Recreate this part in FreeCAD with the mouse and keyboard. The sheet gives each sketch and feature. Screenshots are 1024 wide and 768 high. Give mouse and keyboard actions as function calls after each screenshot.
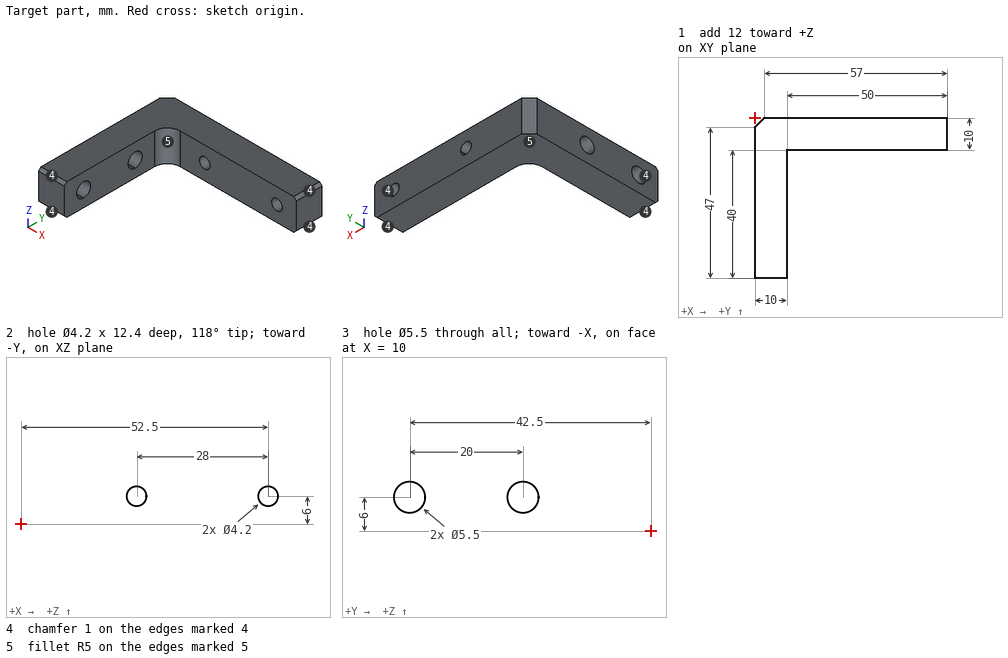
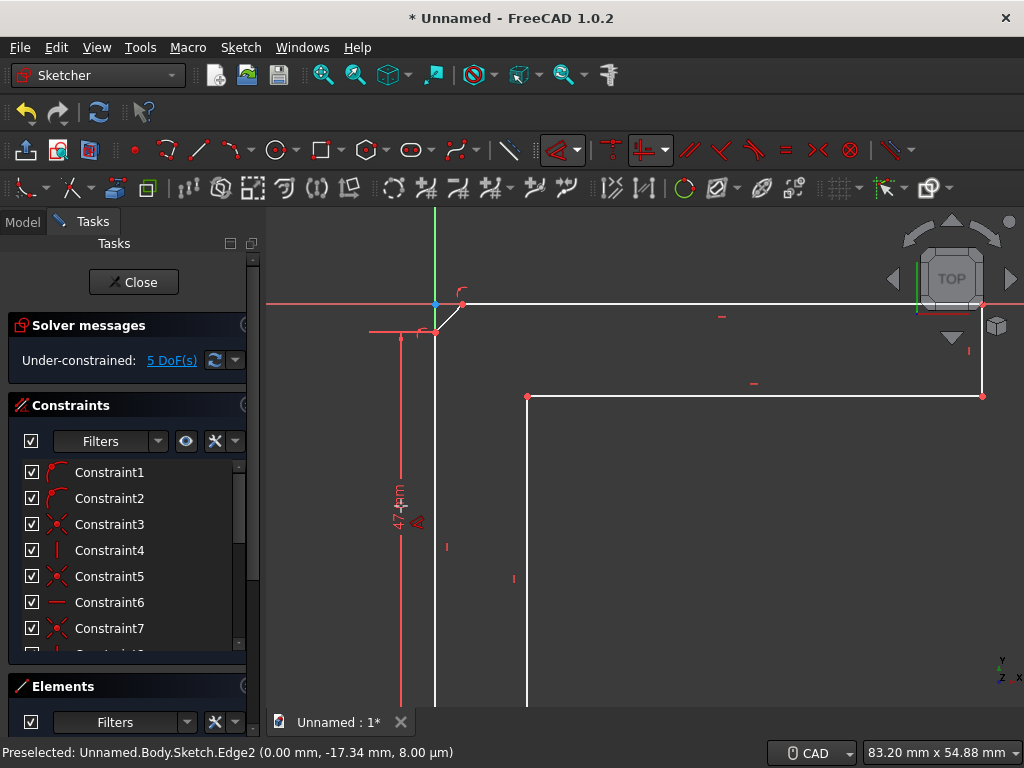
scroll(308, 305, down, 2)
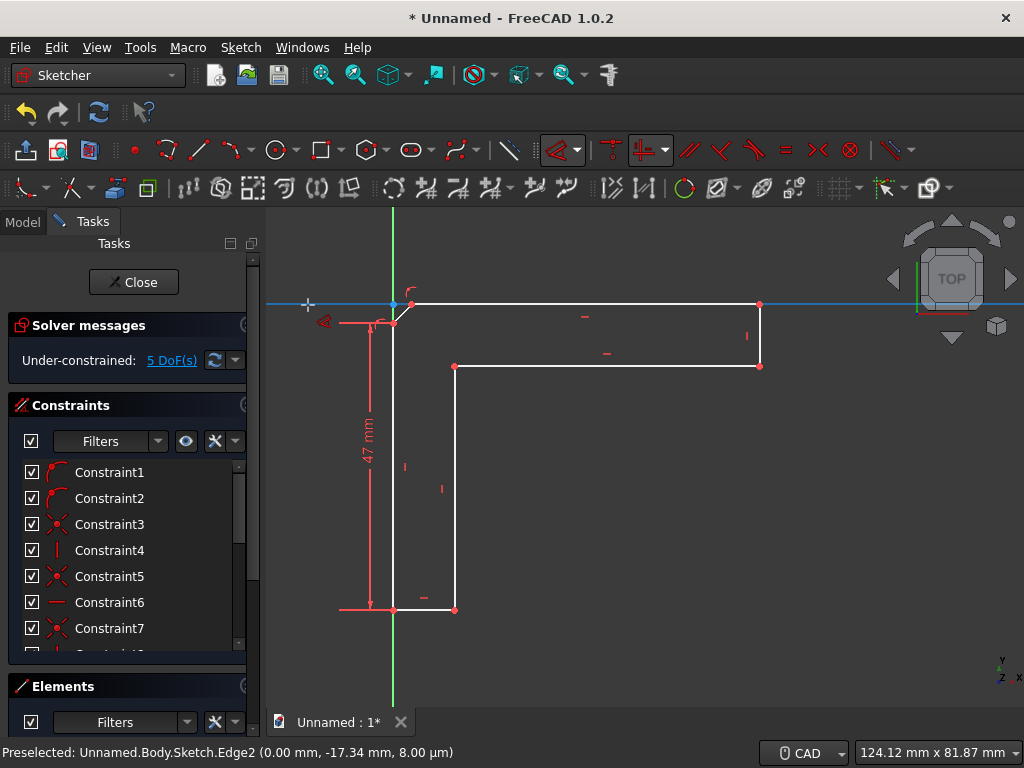
click(412, 610)
click(424, 644)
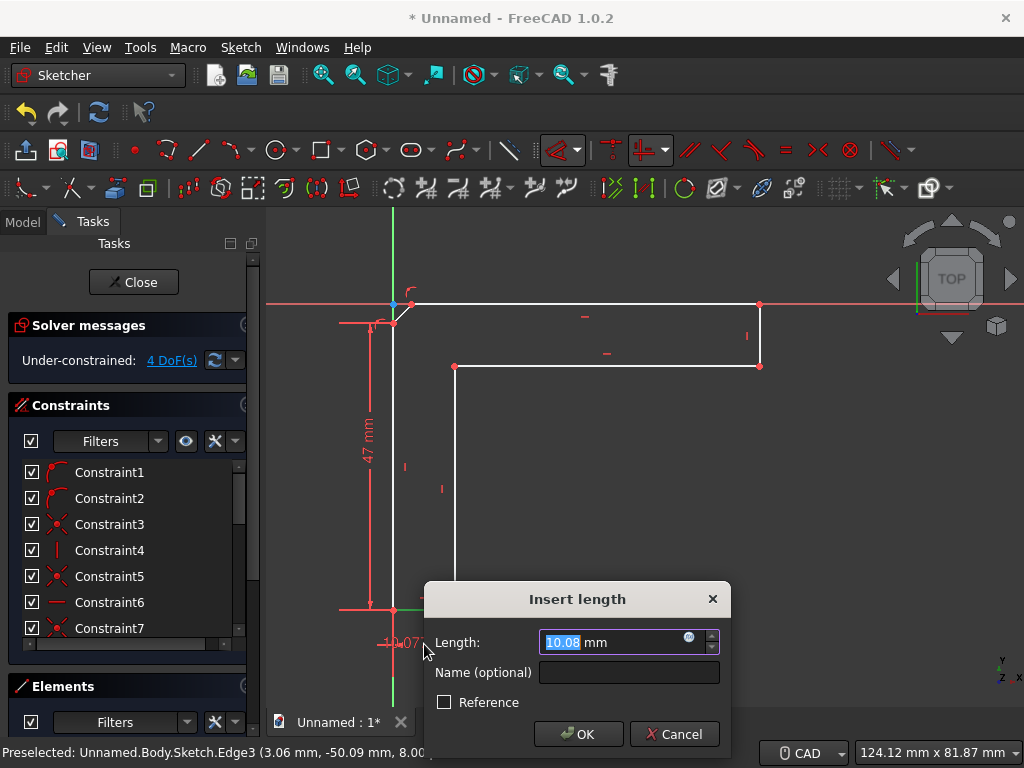
text(10)
key(Return)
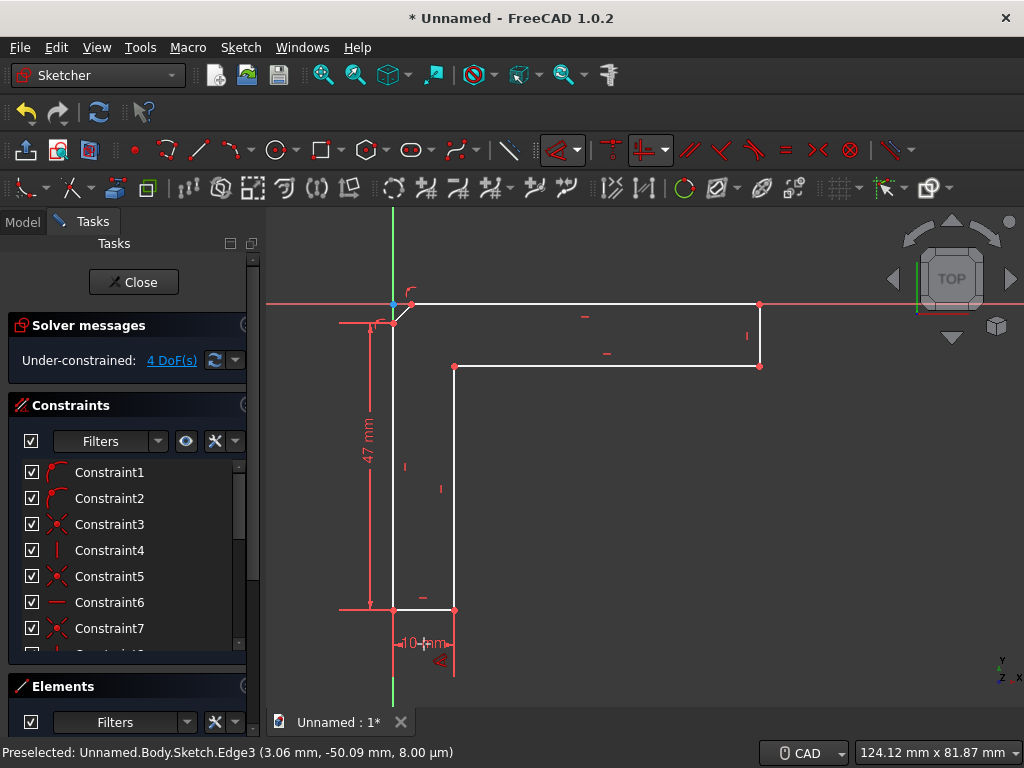
click(454, 537)
click(420, 488)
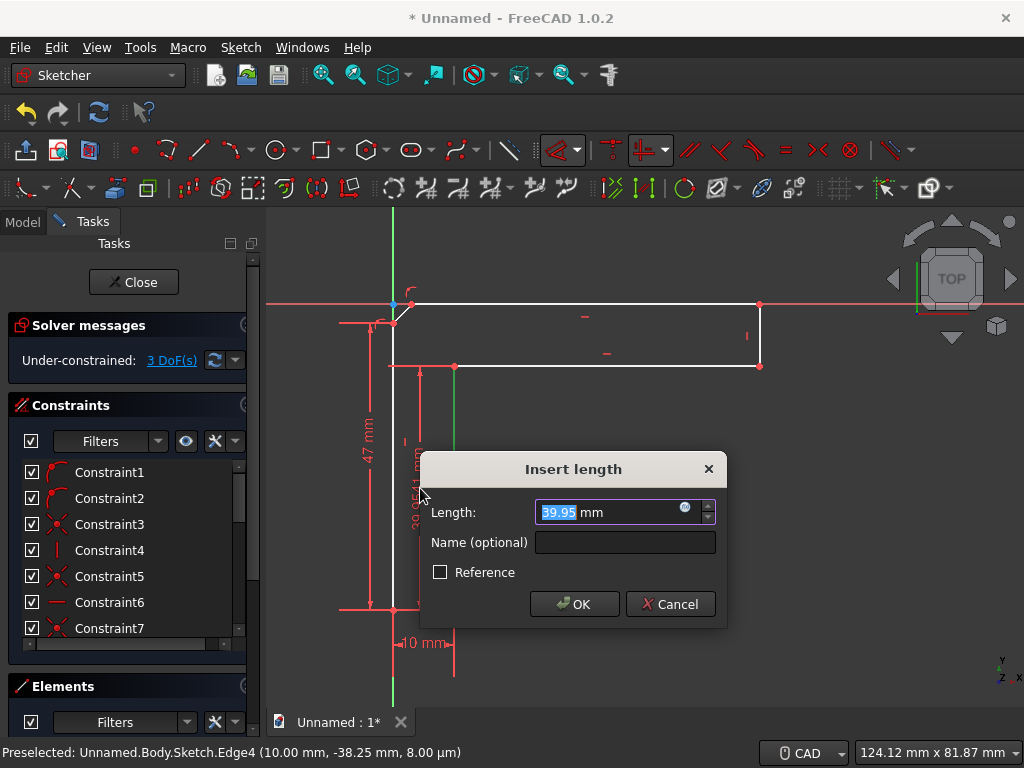
text(40)
key(Return)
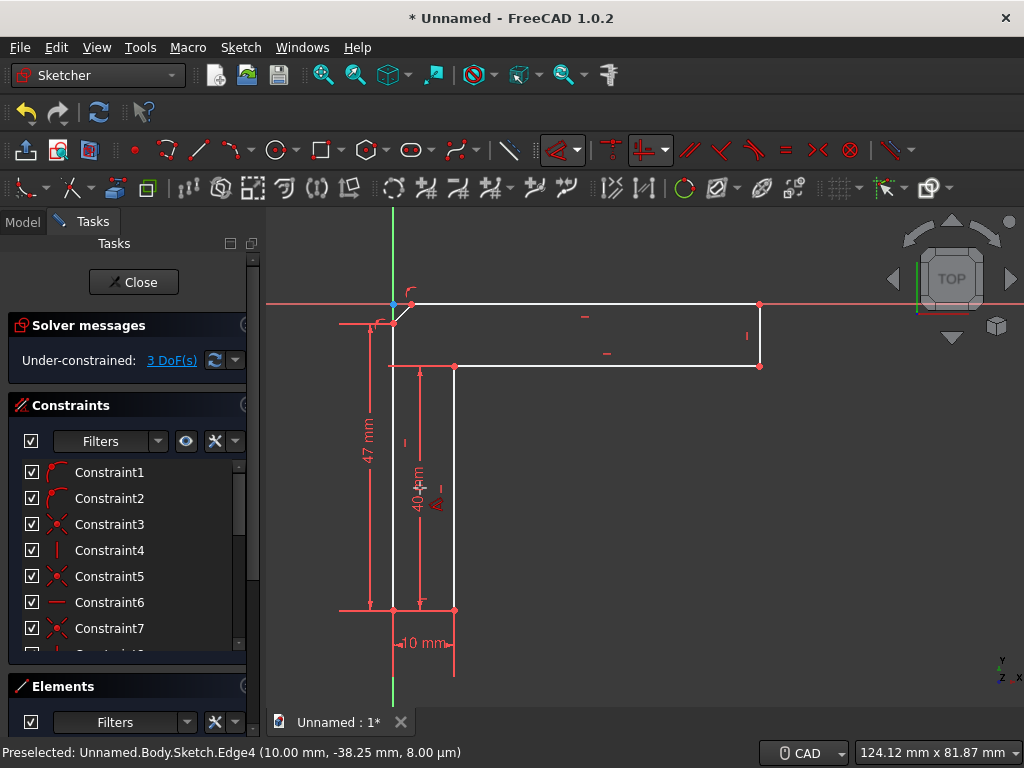
click(546, 366)
click(607, 332)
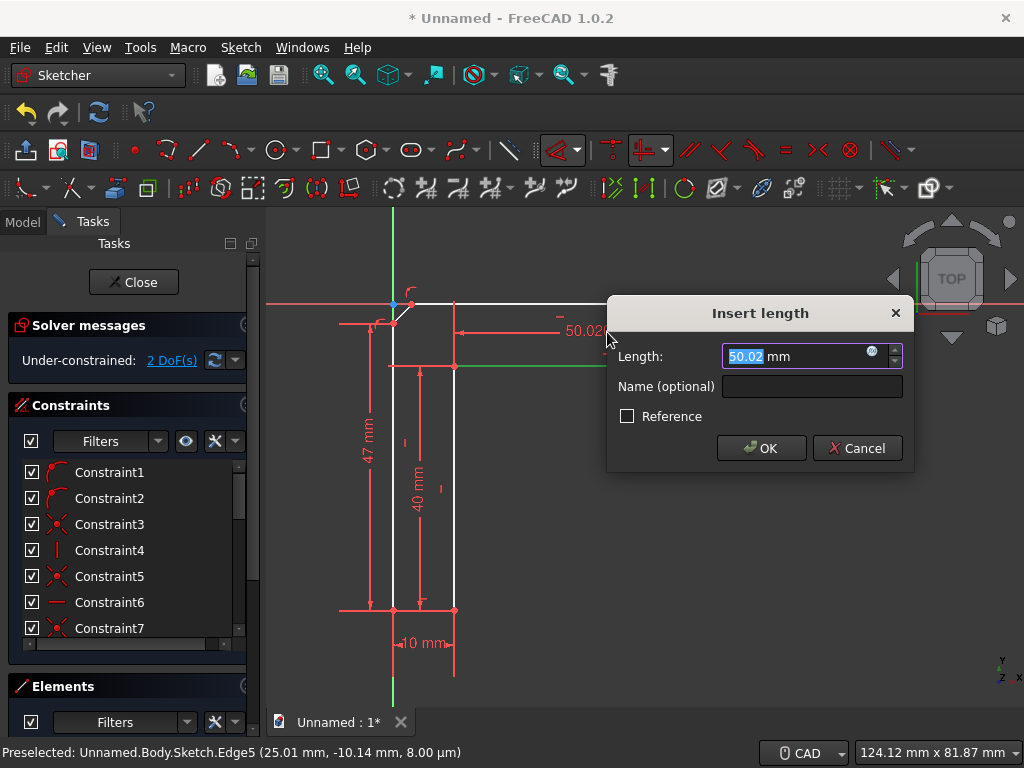
text(50)
key(Return)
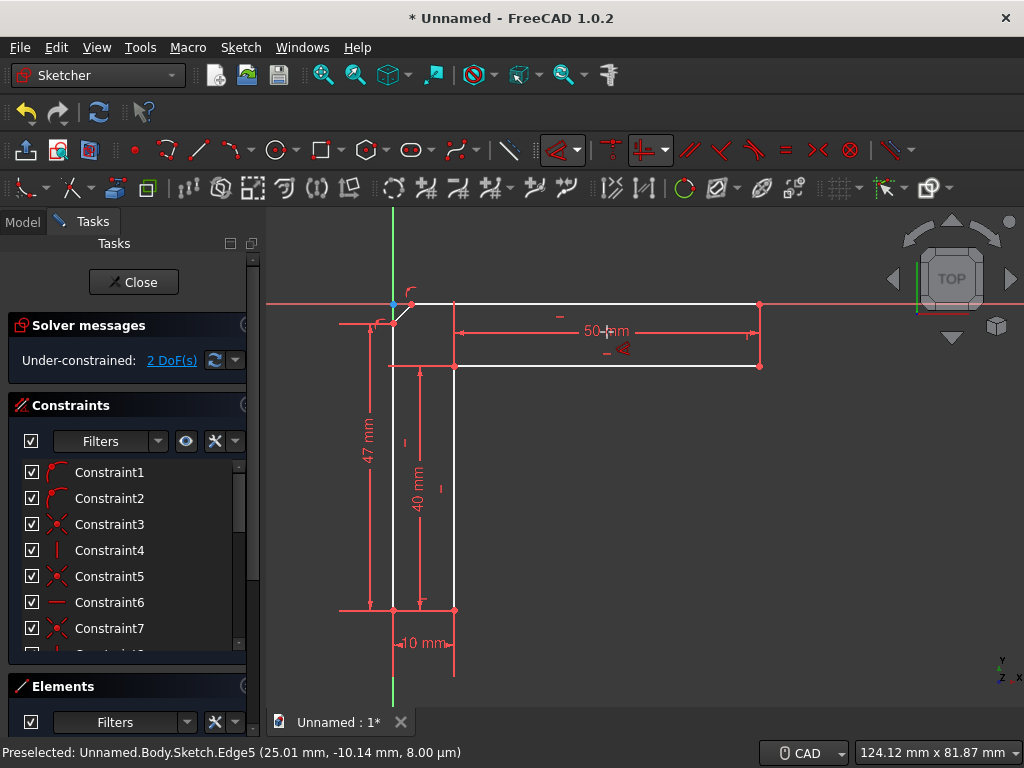
click(760, 348)
click(794, 335)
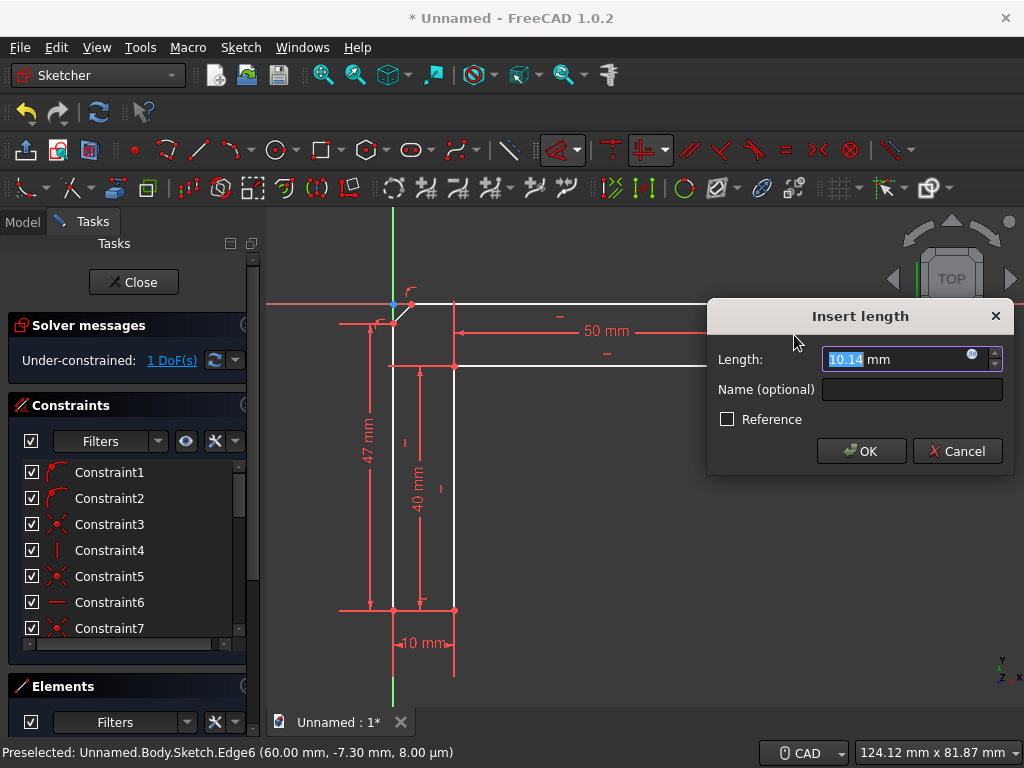
text(10)
key(Return)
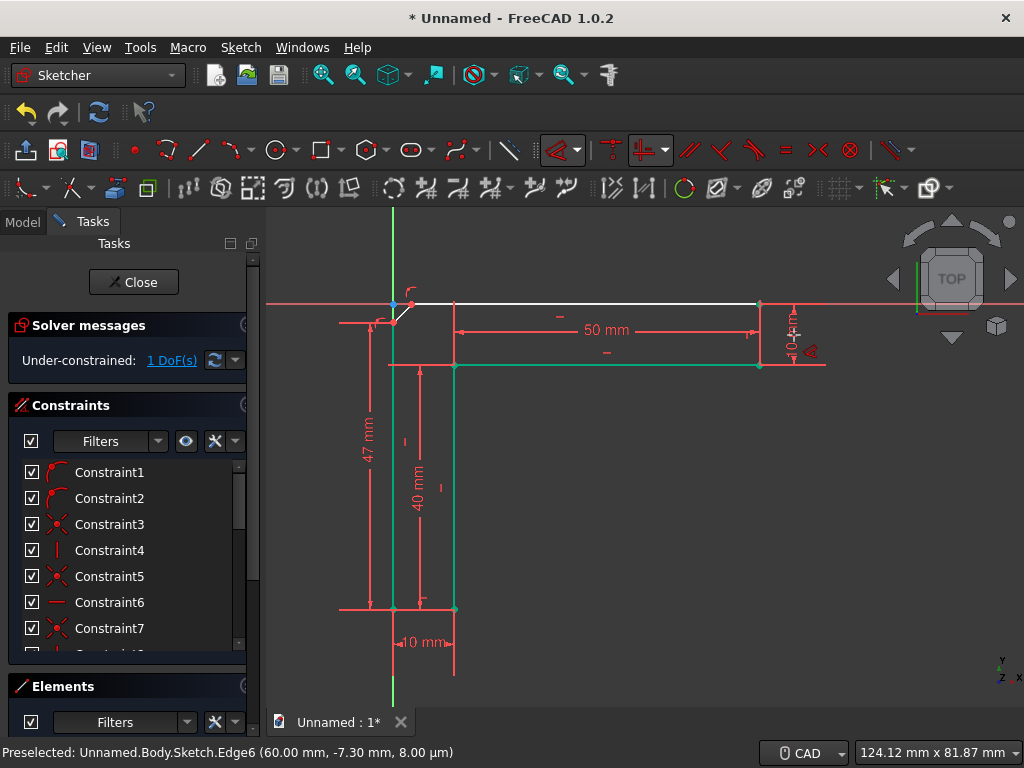
click(655, 304)
click(586, 270)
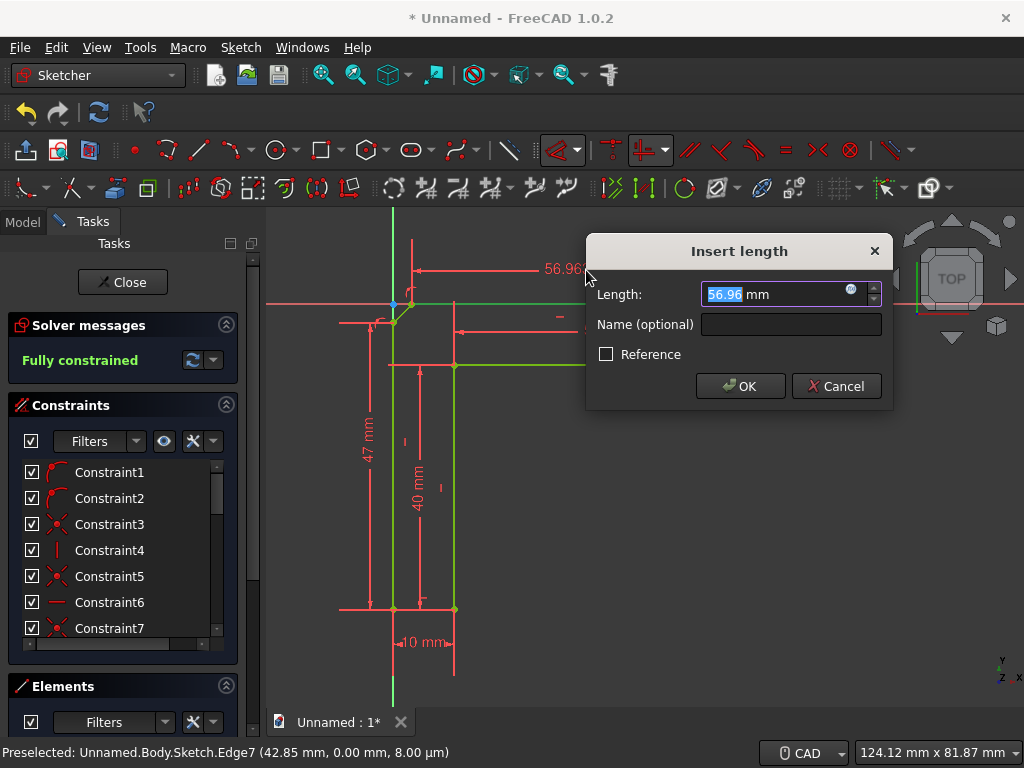
text(57)
key(Return)
key(Escape)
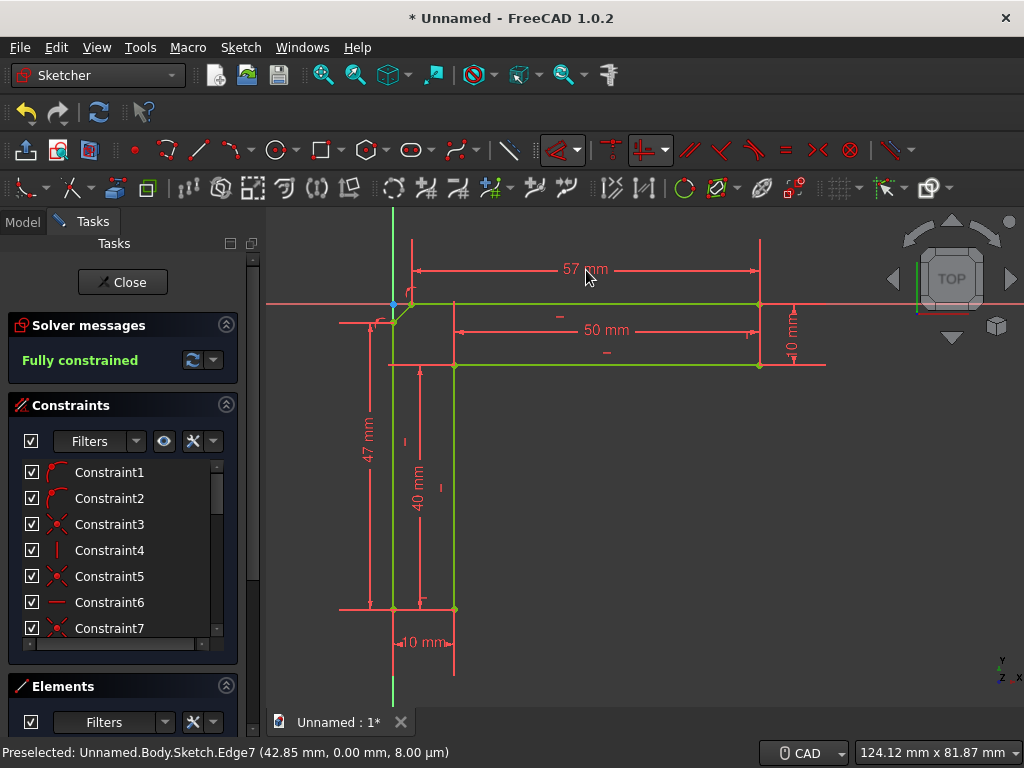
click(123, 282)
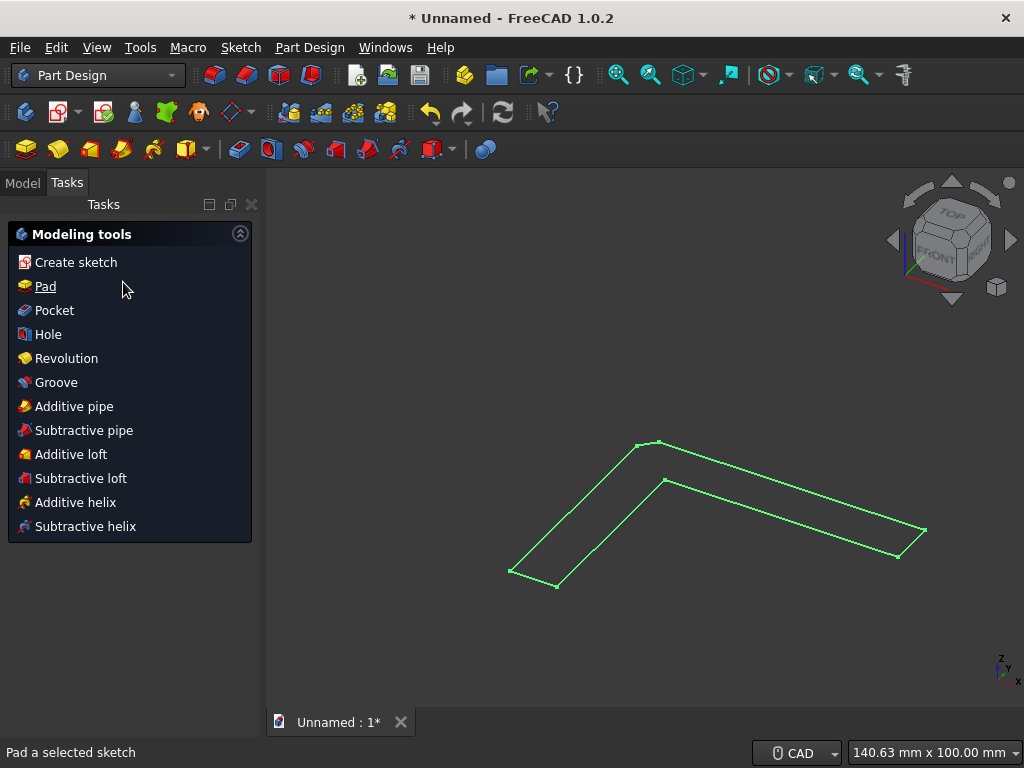
click(26, 150)